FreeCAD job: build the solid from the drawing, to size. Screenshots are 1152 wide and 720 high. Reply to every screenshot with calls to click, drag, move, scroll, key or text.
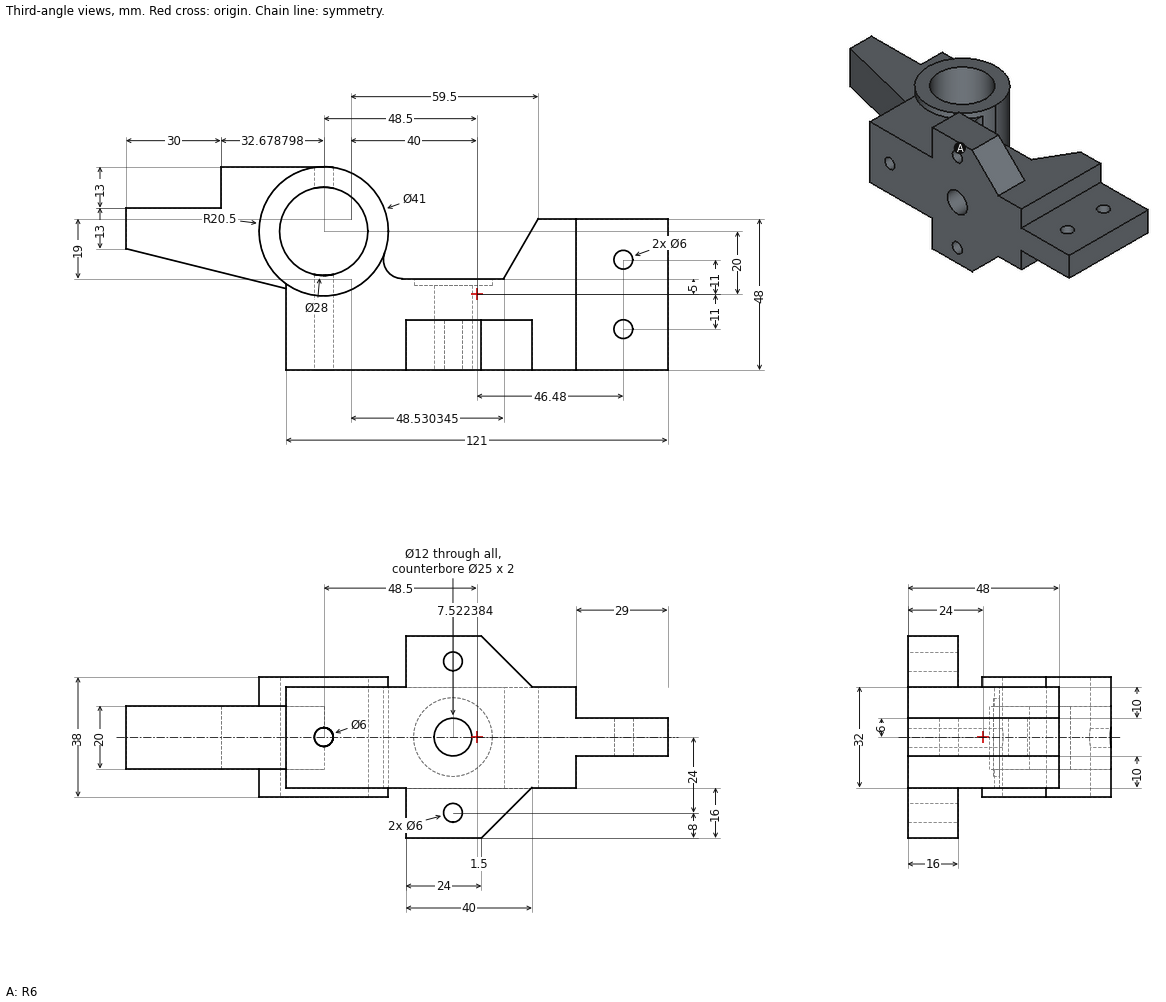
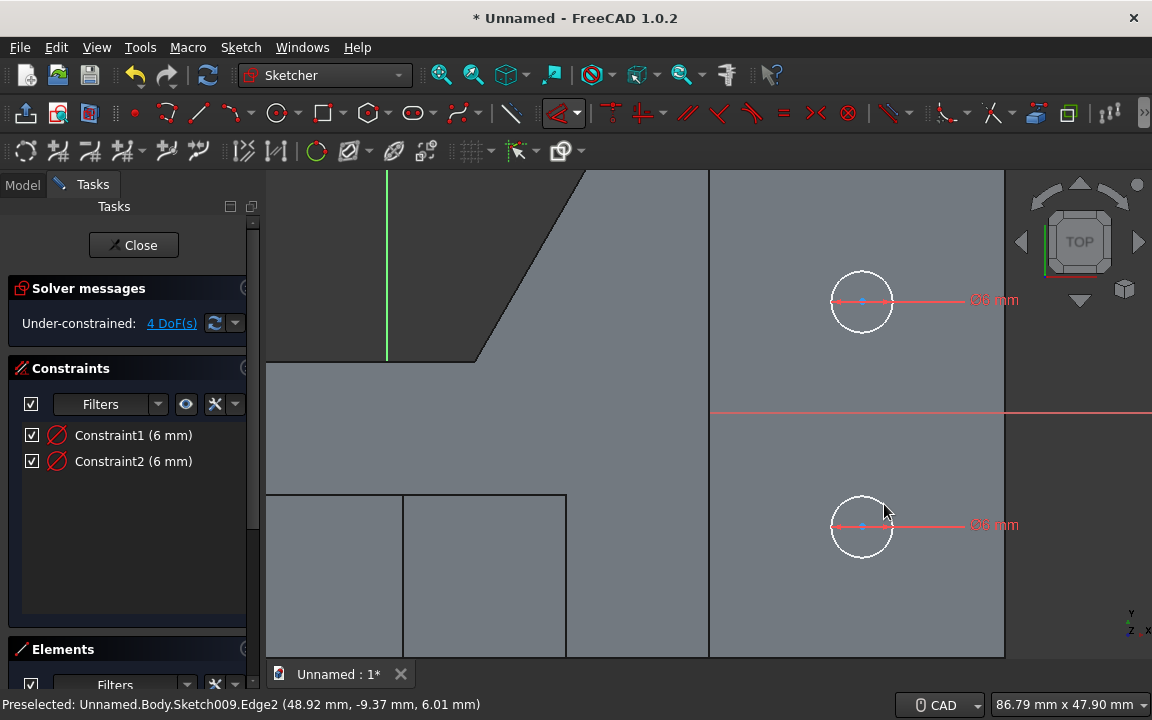
click(862, 302)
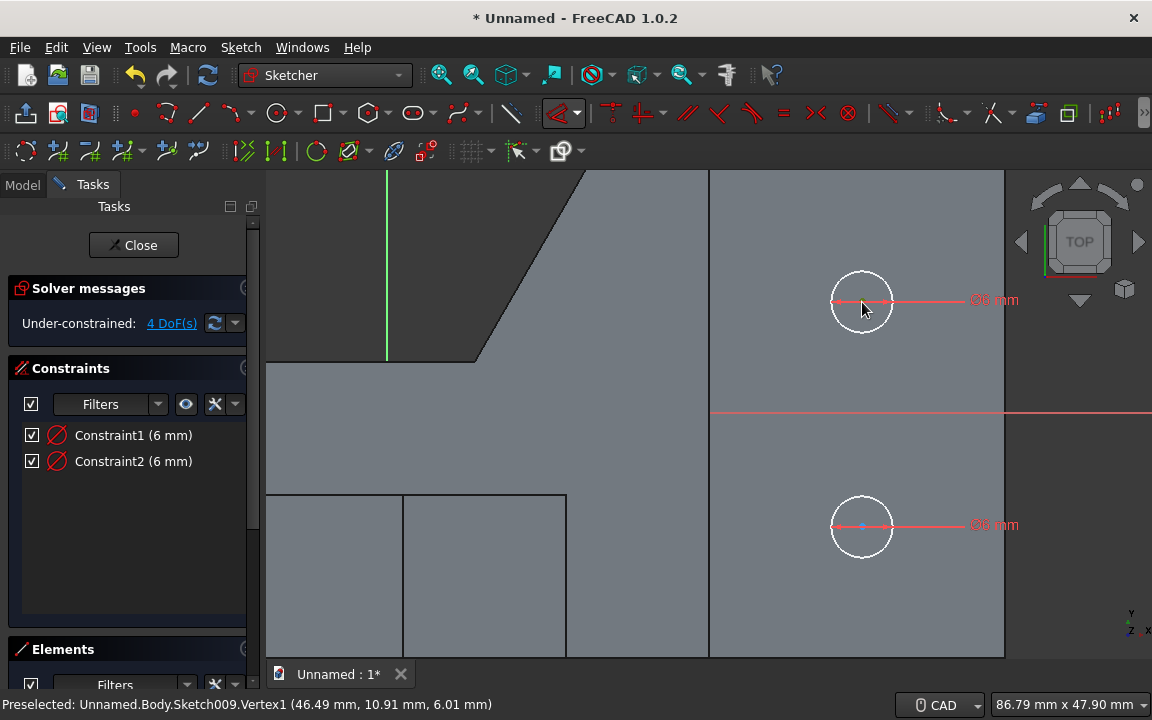
click(862, 527)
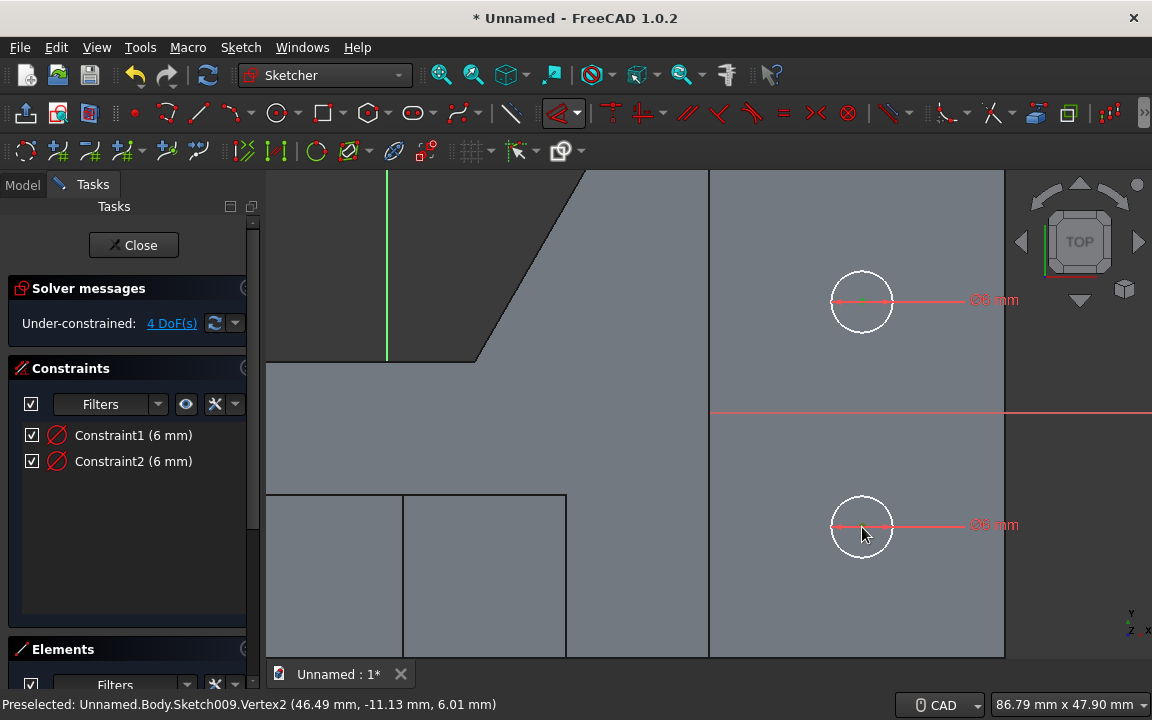
key(v)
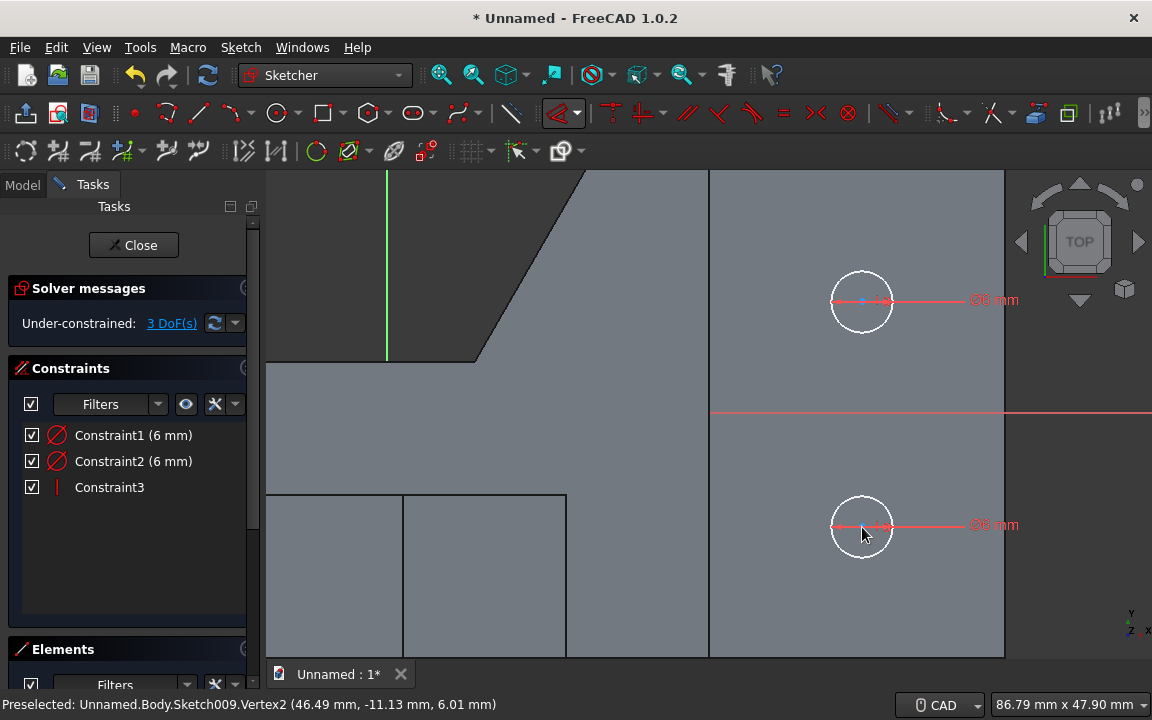
click(862, 302)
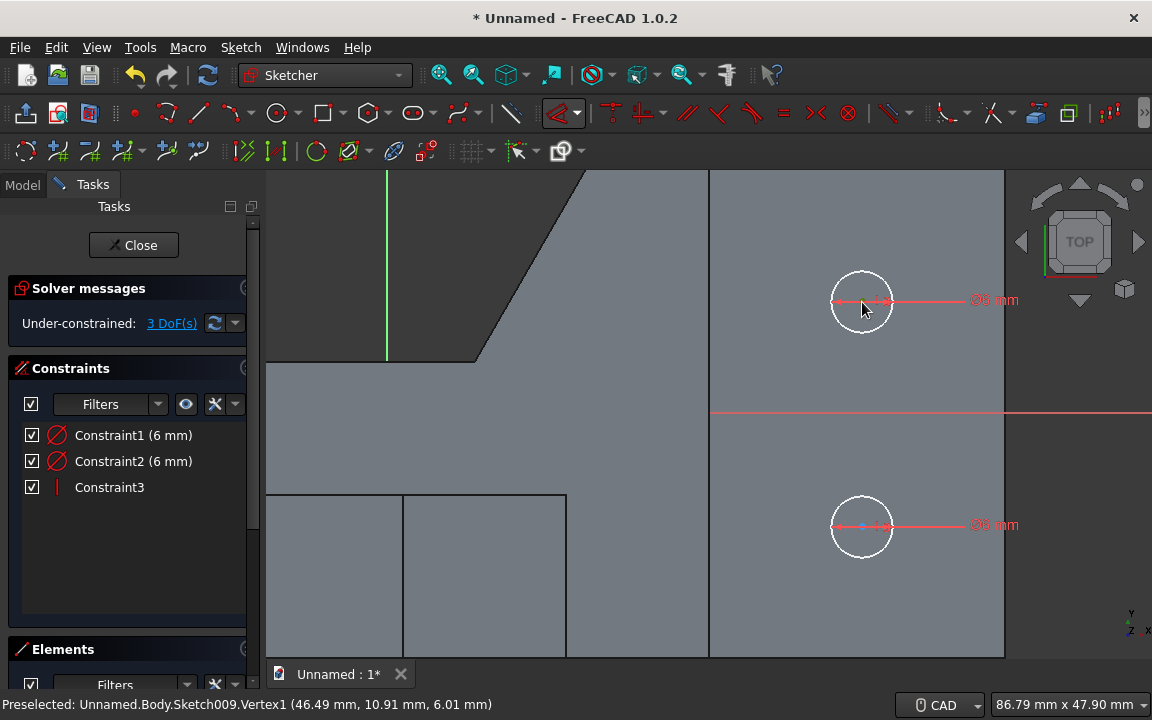
click(580, 114)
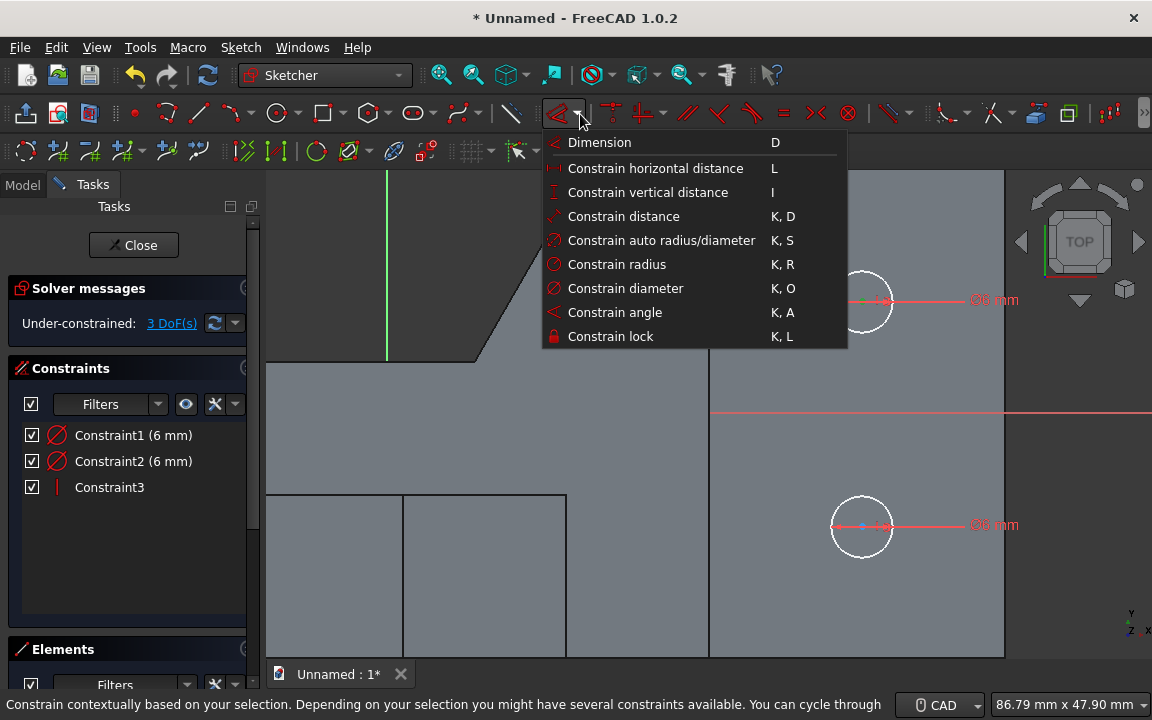
click(695, 192)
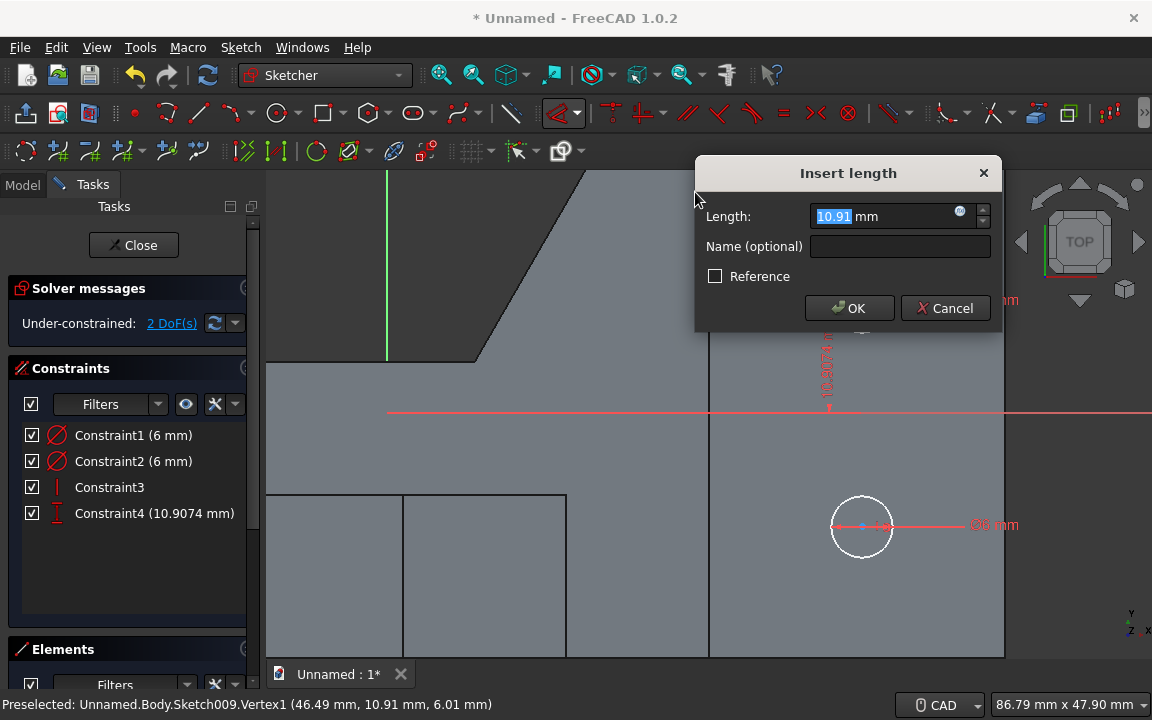
text(11)
key(Return)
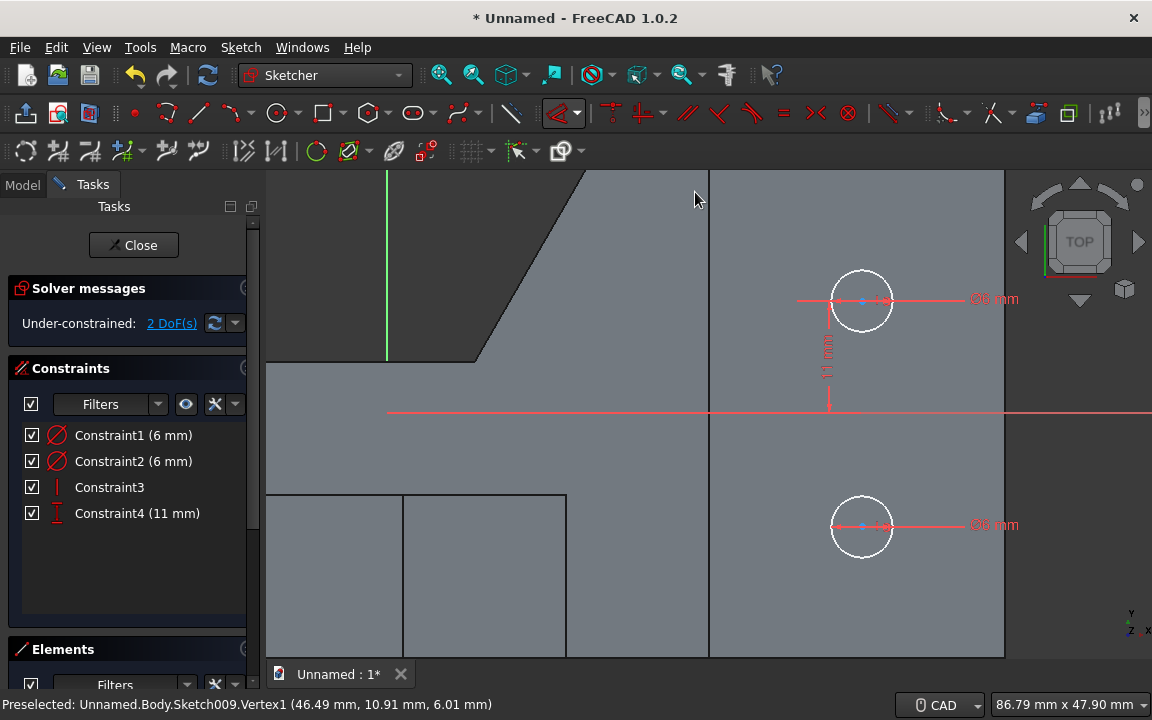
click(862, 527)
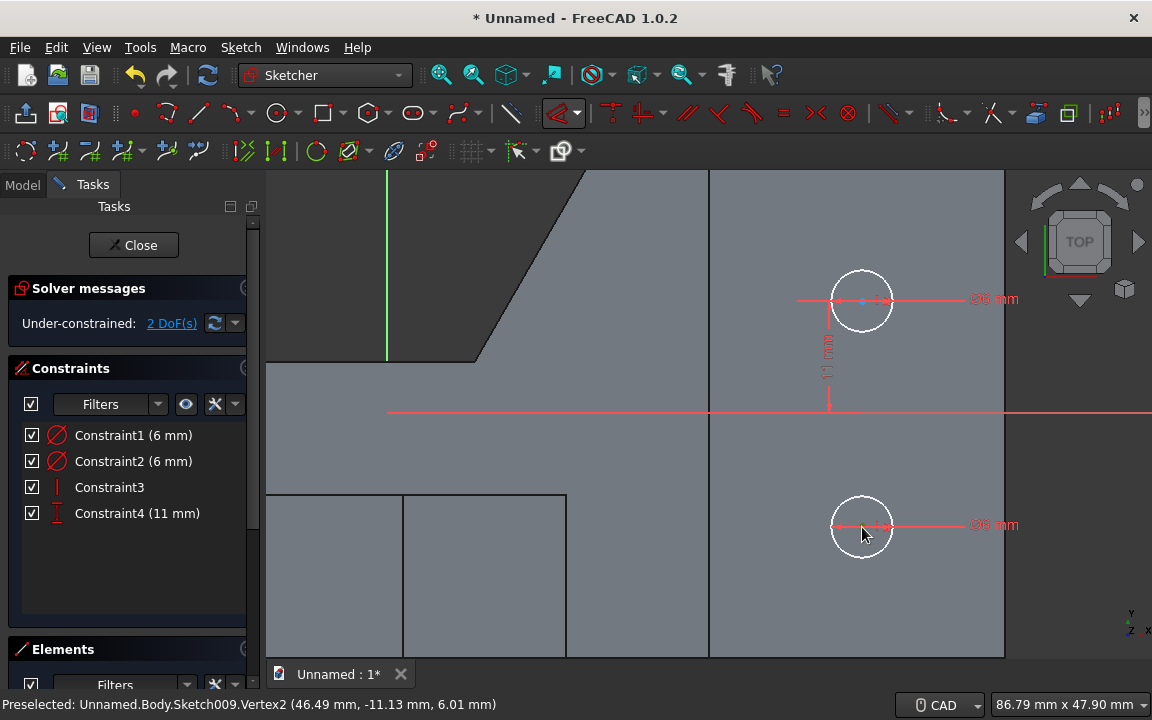
key(i)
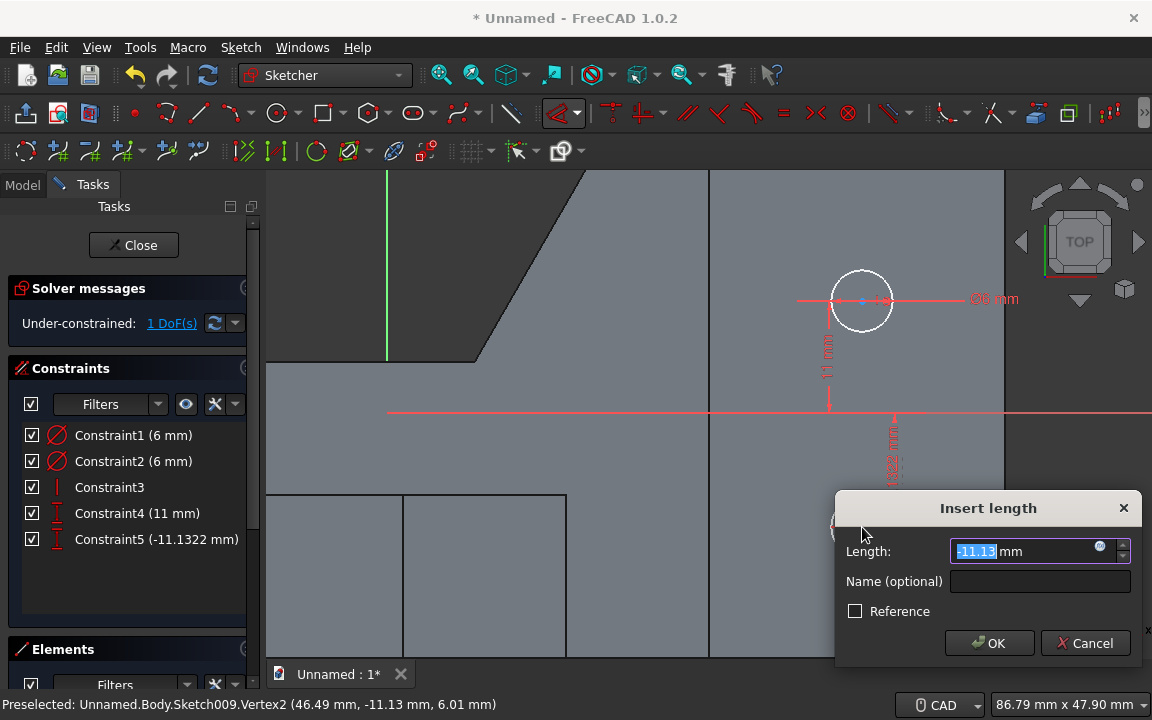
text(-11)
key(Return)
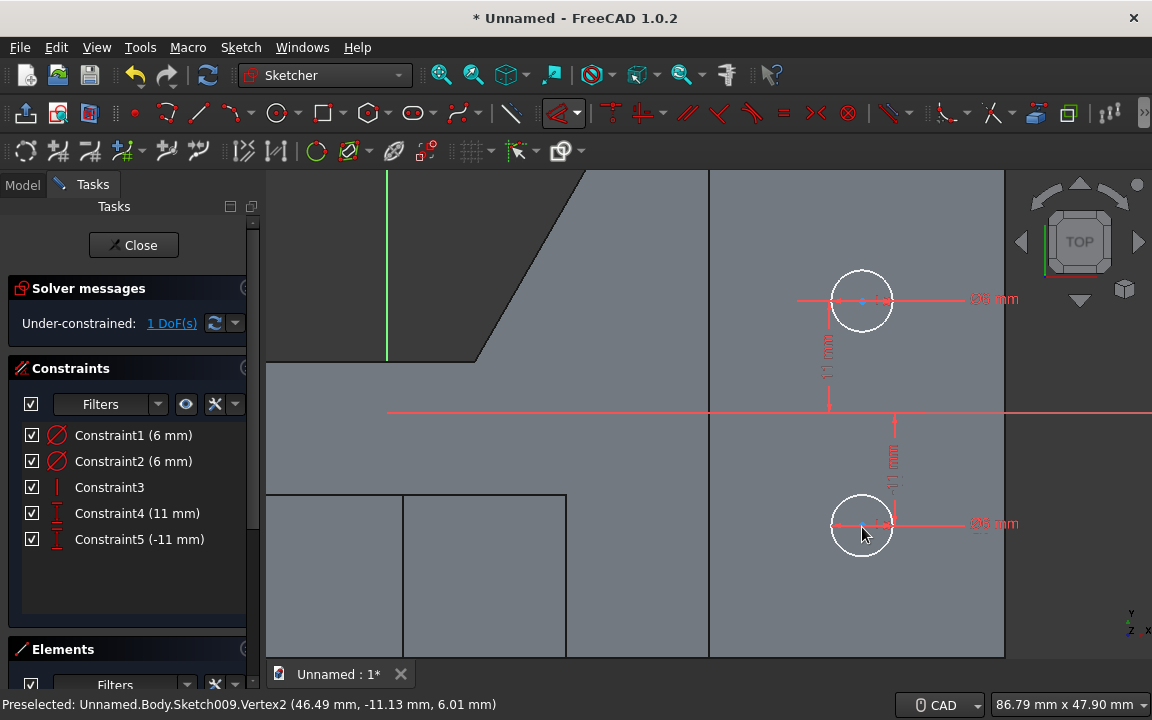
click(862, 301)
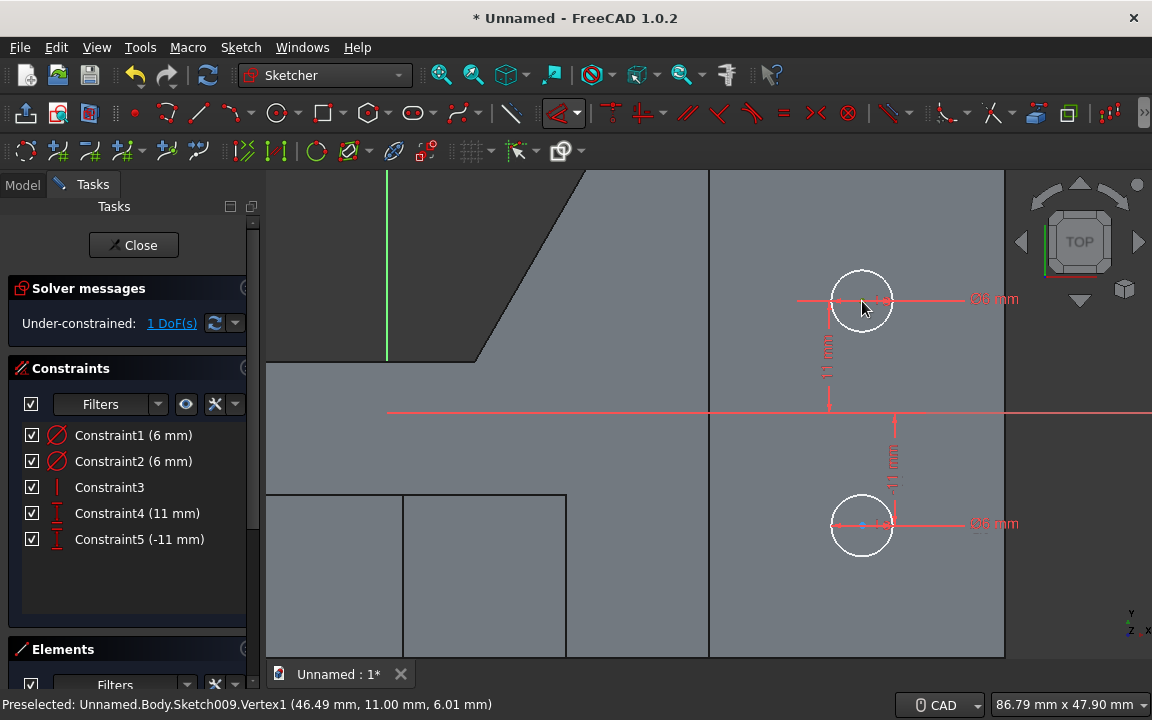
key(l)